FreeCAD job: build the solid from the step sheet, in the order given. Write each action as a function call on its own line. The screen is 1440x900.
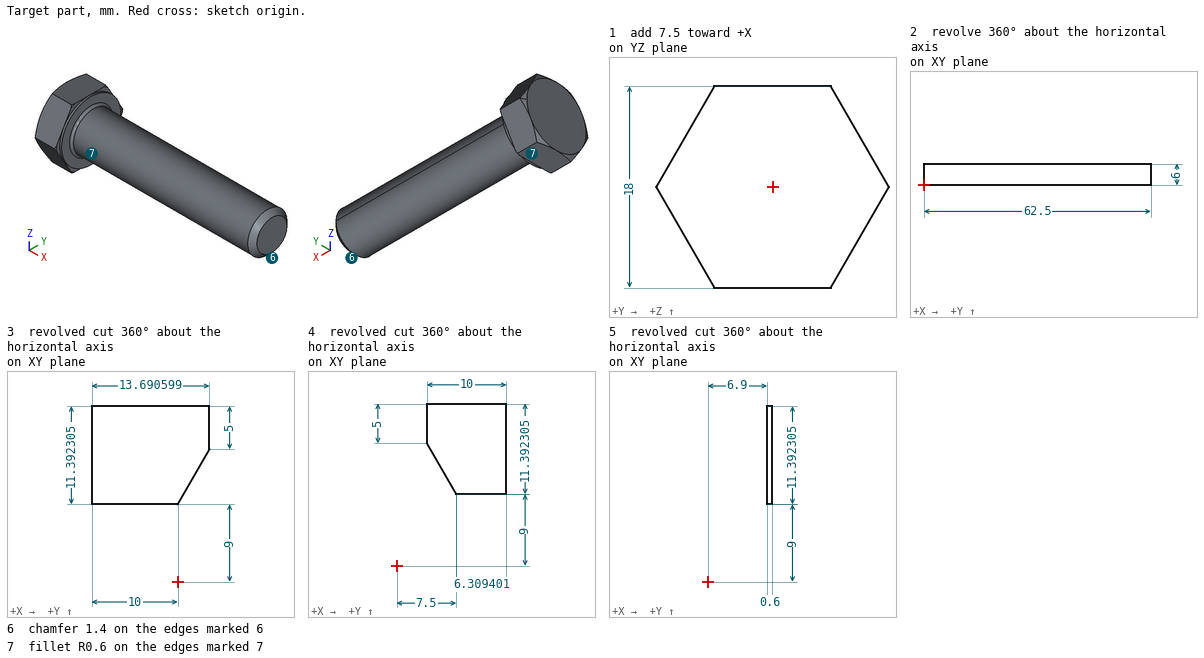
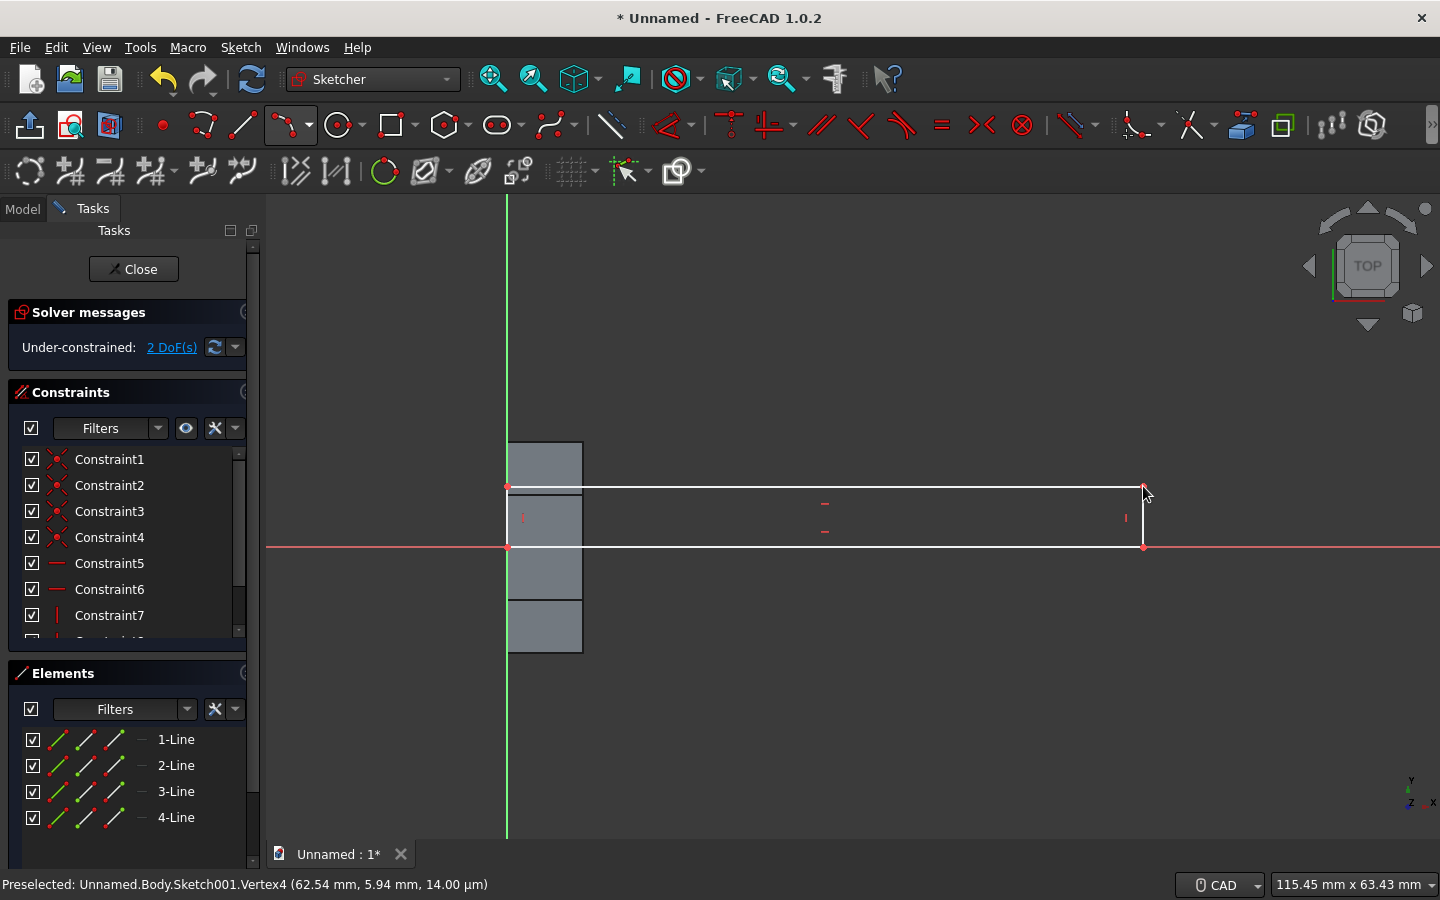
click(666, 126)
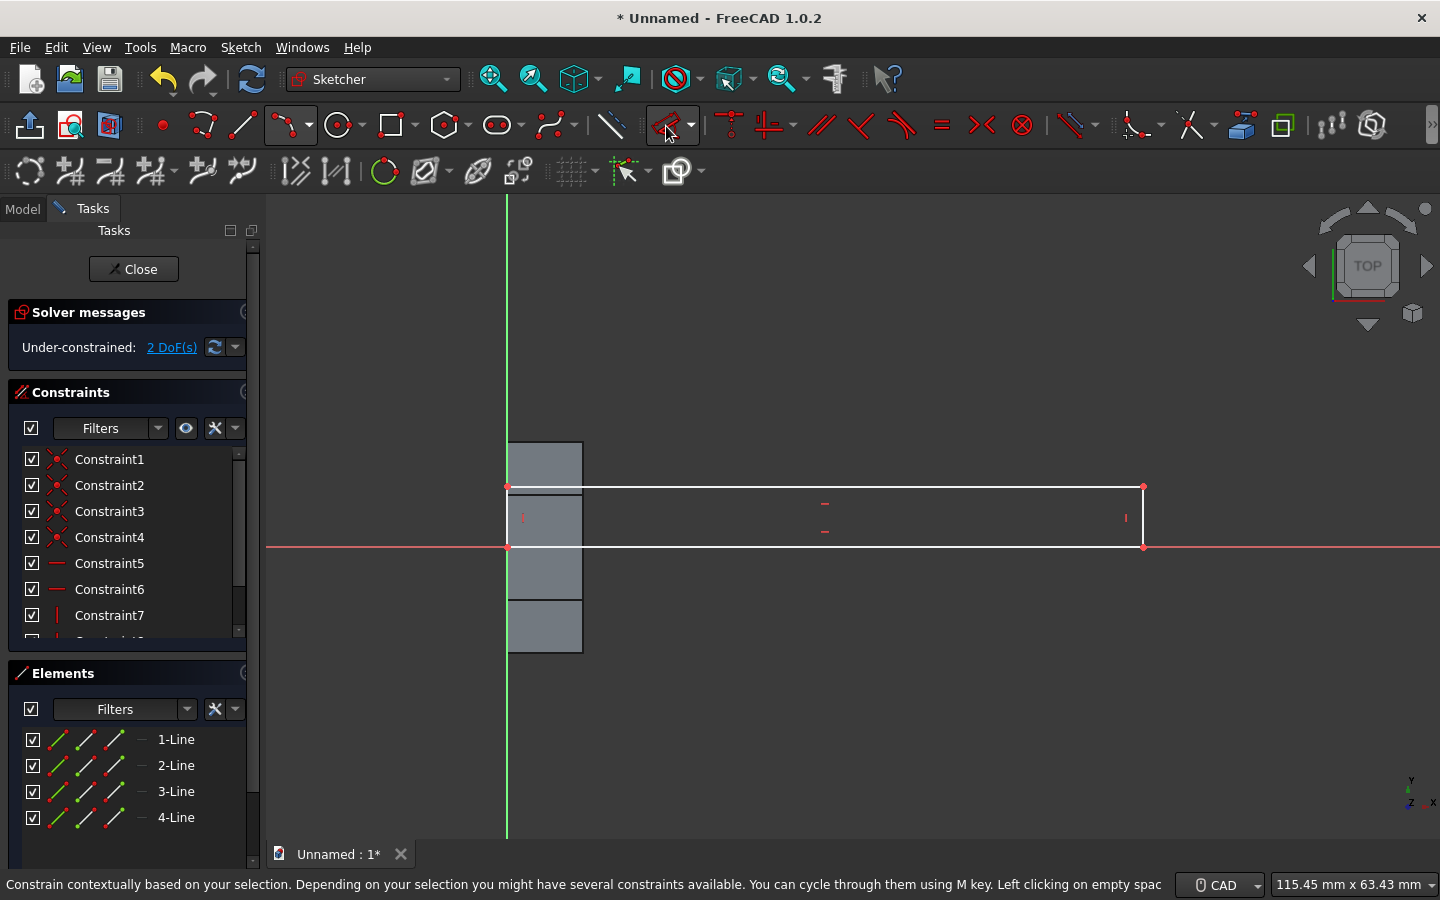
click(1143, 529)
click(1177, 517)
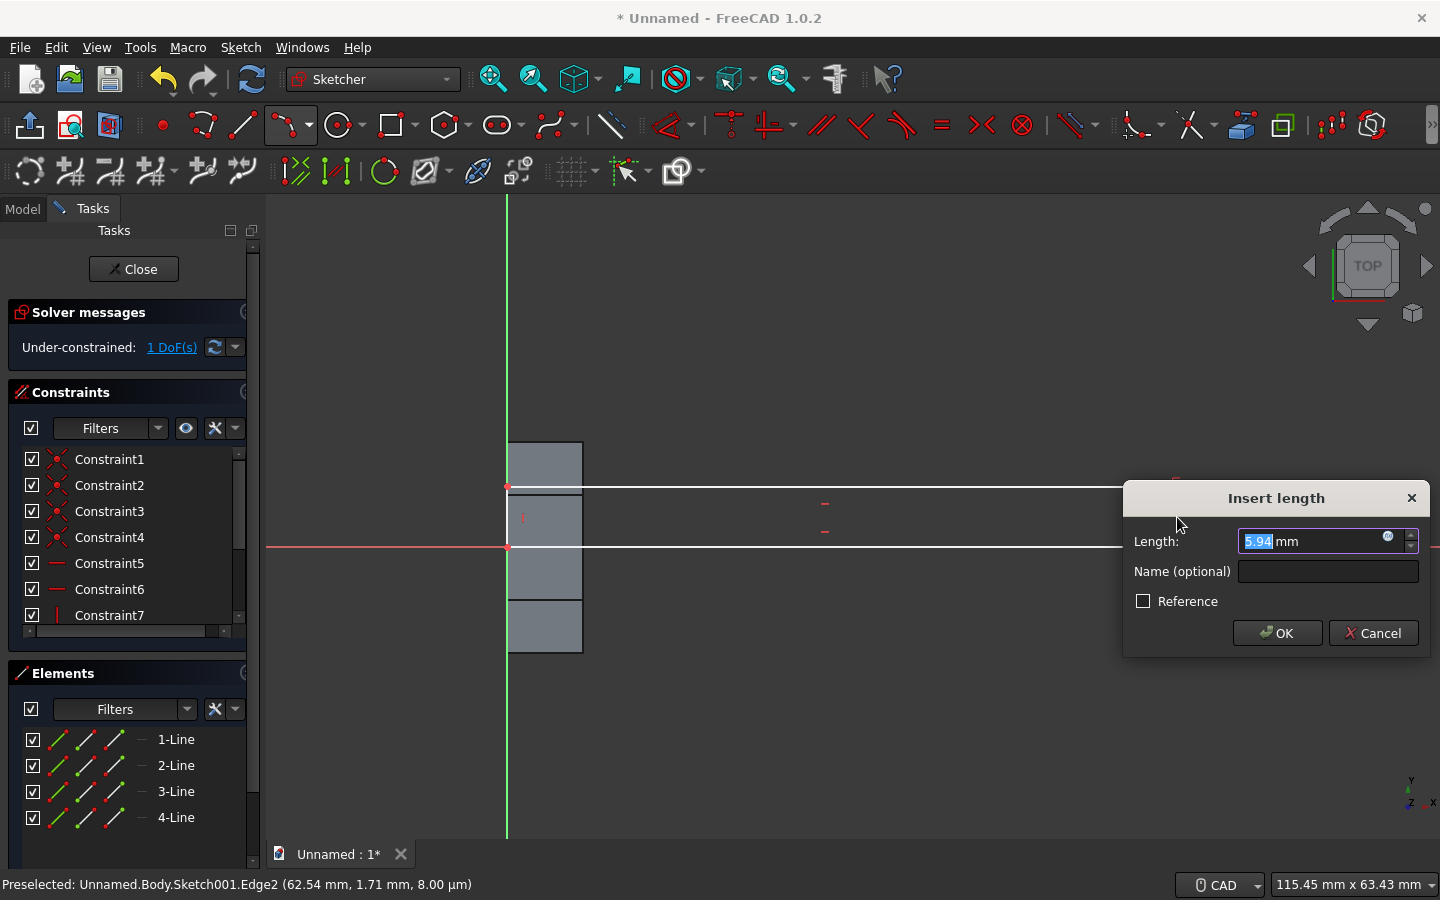
text(6)
key(Return)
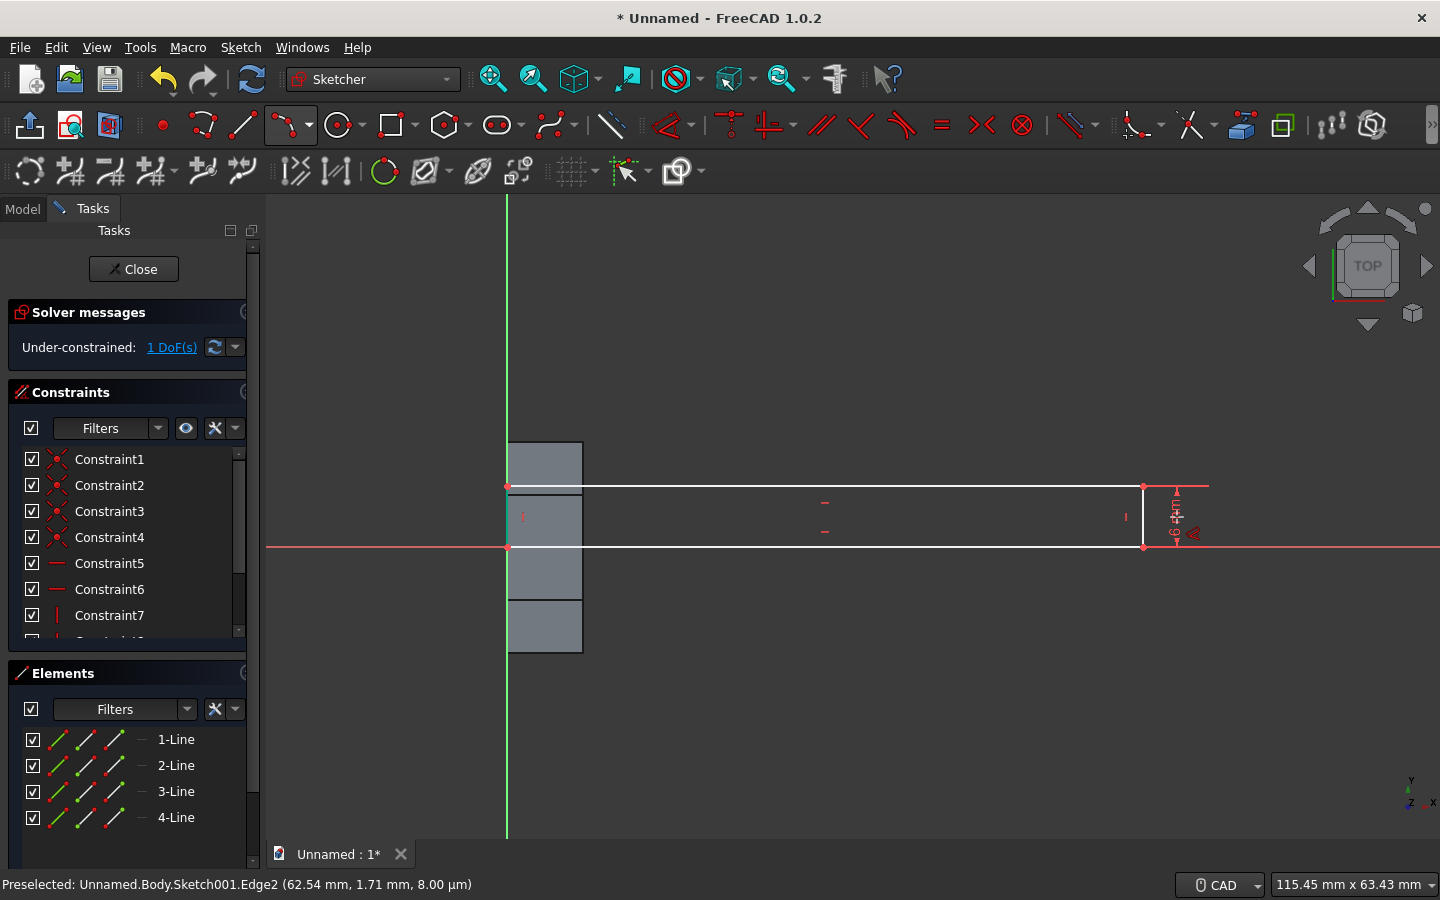
click(698, 547)
click(825, 581)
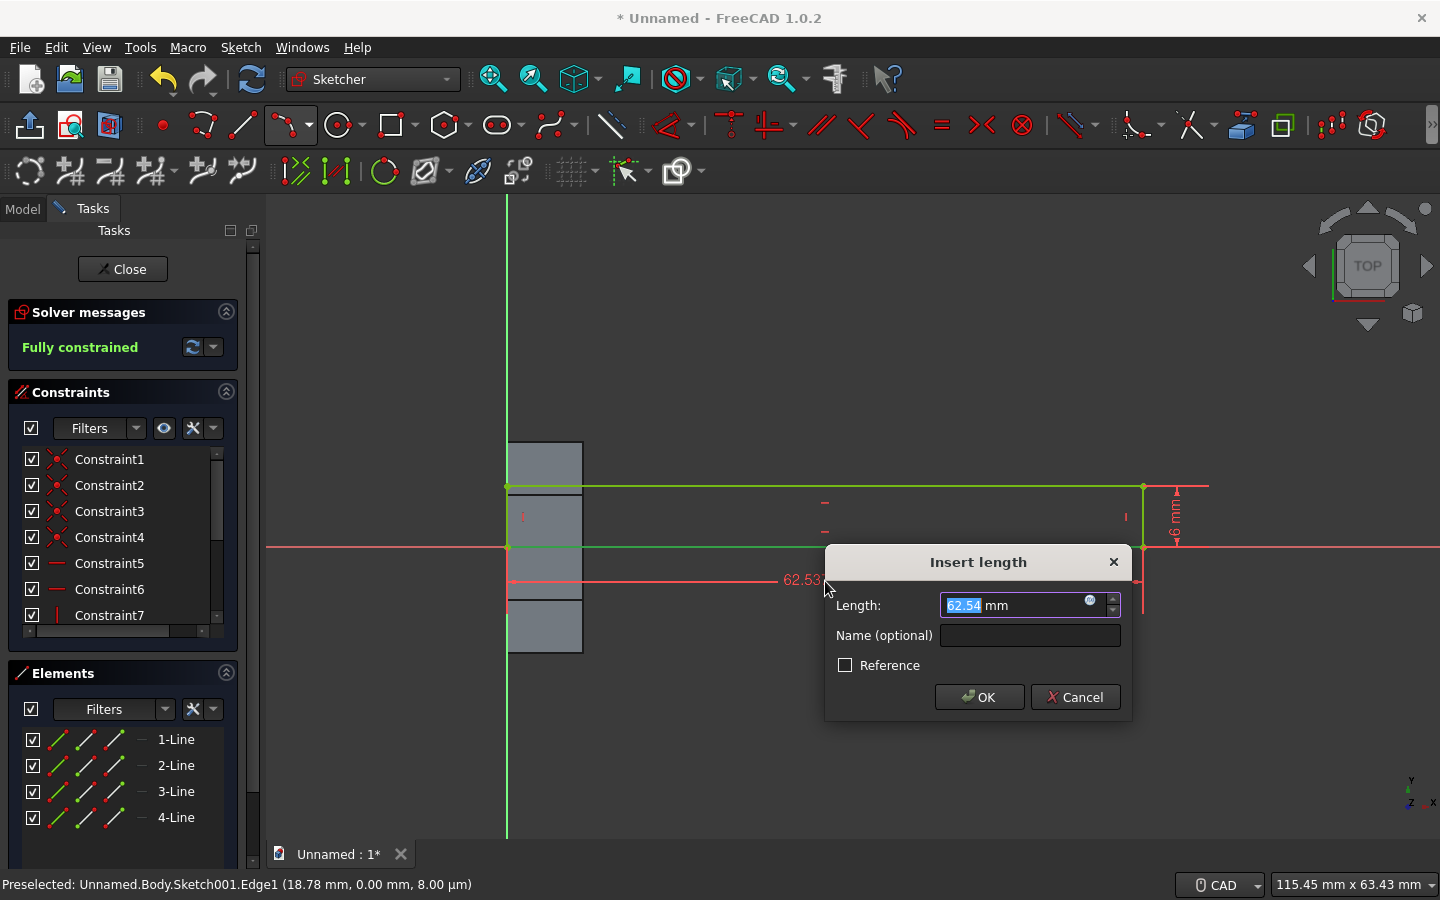
text(62.5)
key(Return)
key(Escape)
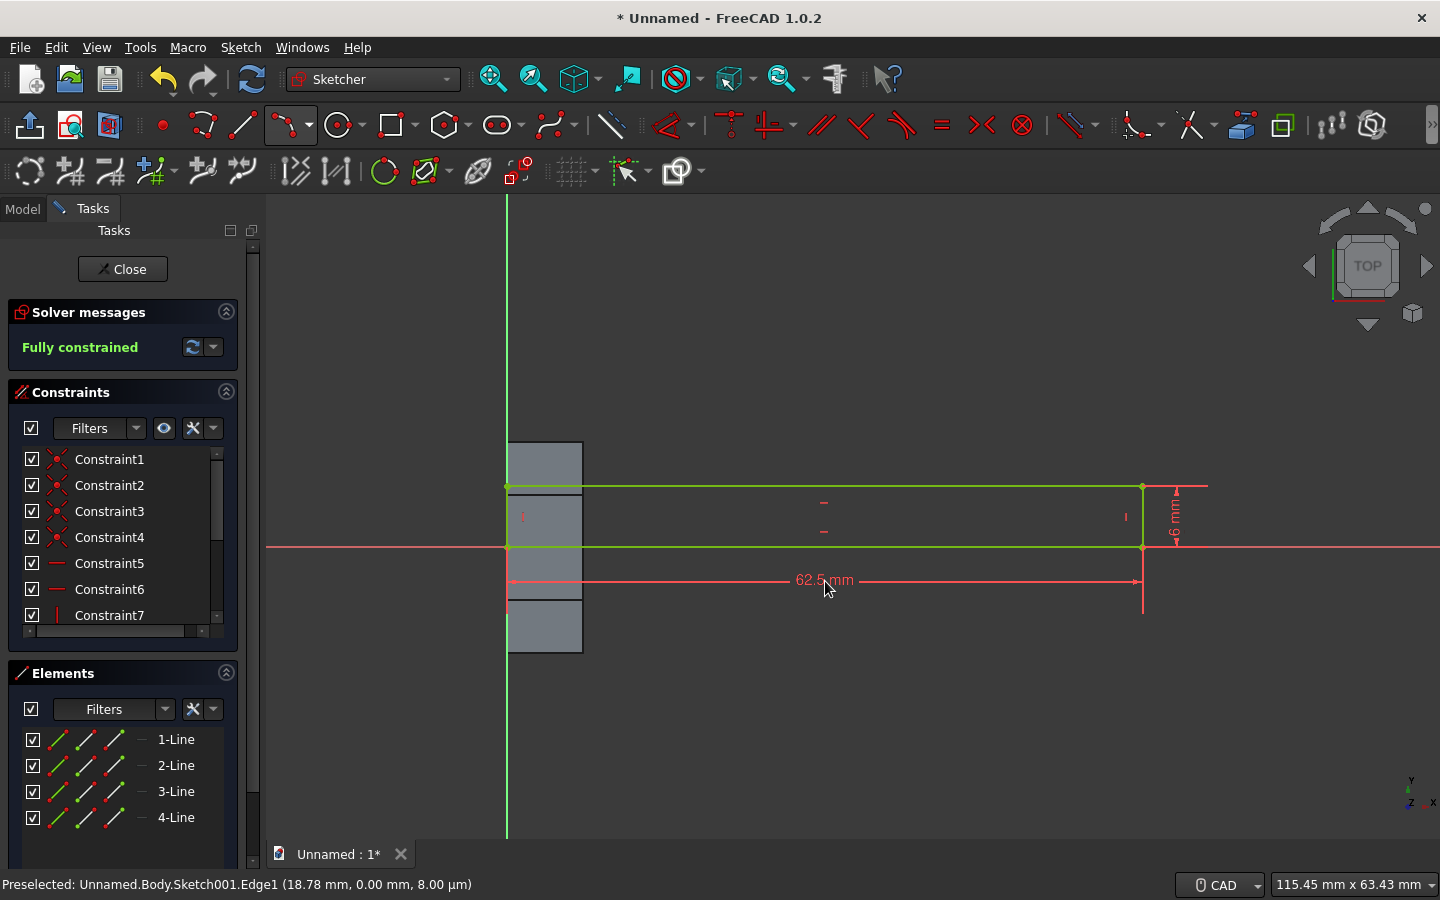
click(123, 269)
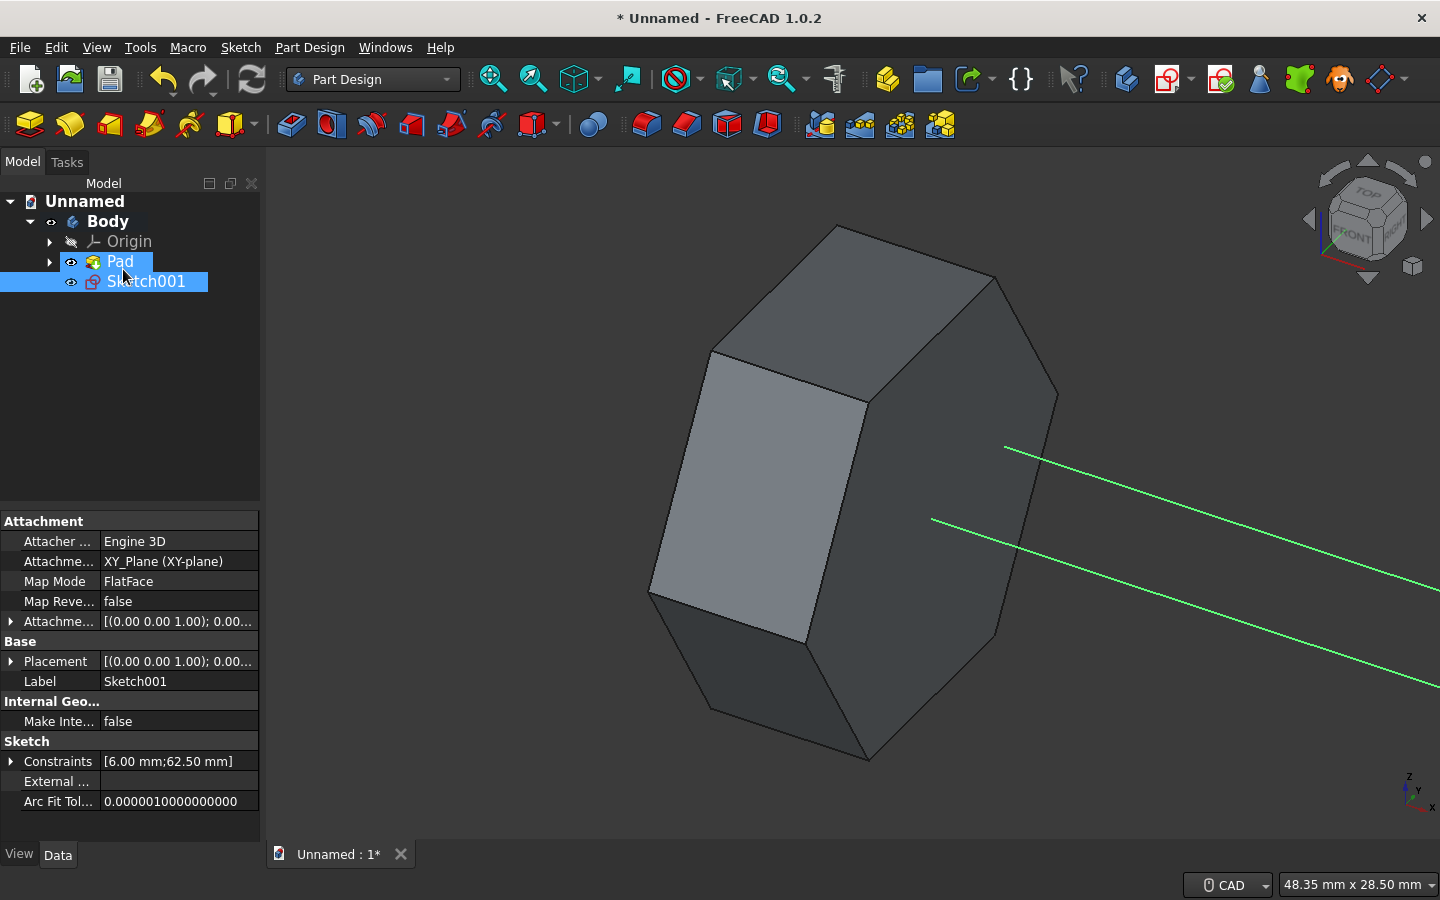
click(70, 124)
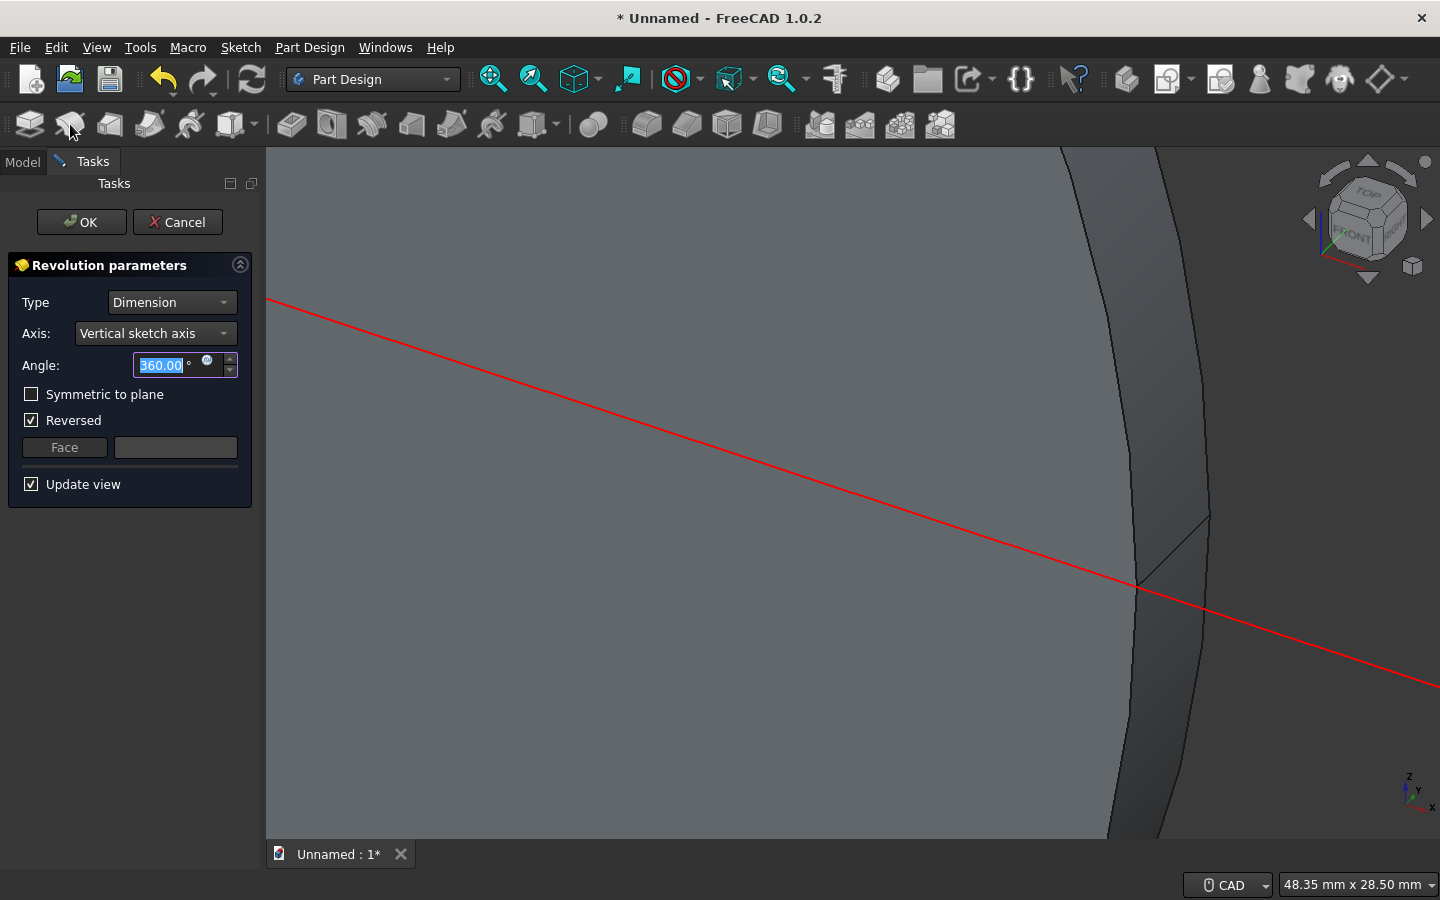
click(156, 334)